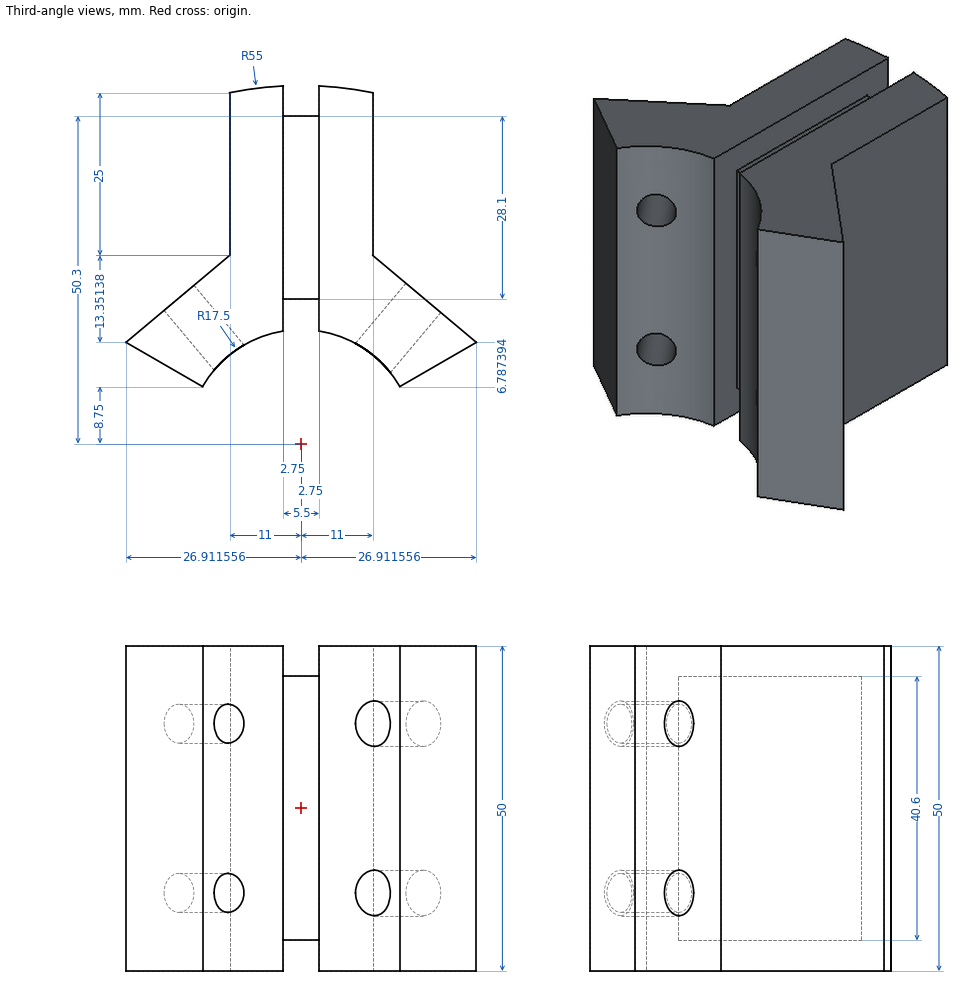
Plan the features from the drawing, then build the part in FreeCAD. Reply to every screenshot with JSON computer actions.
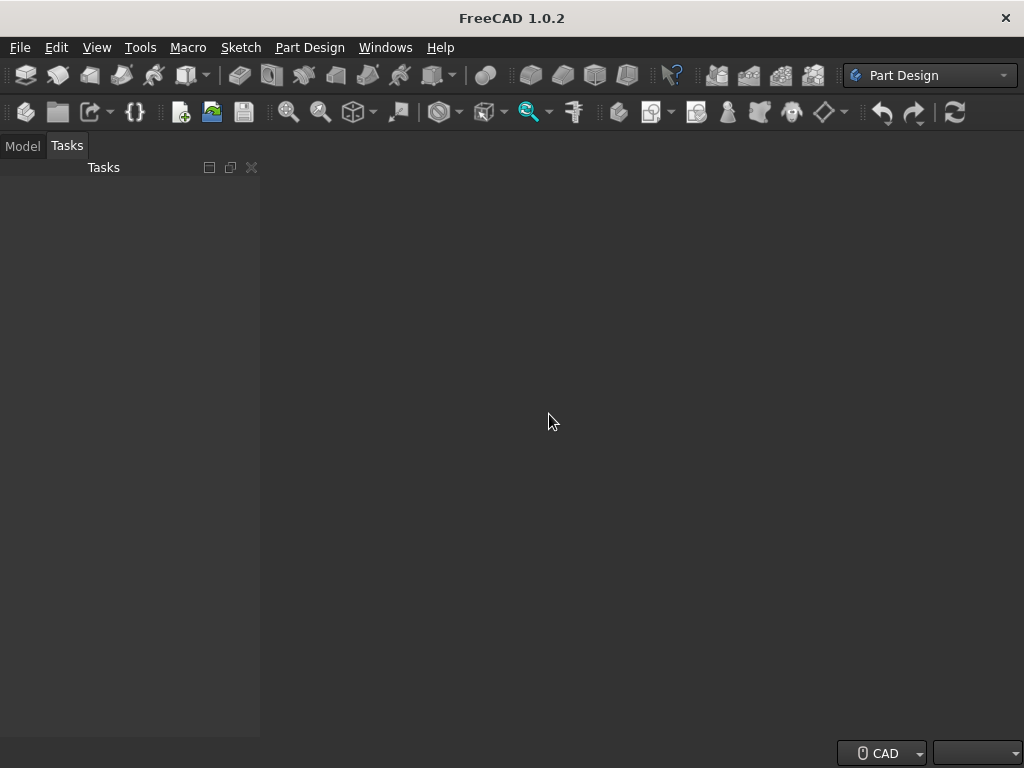
{"action": "left_click", "coordinate": [180, 112]}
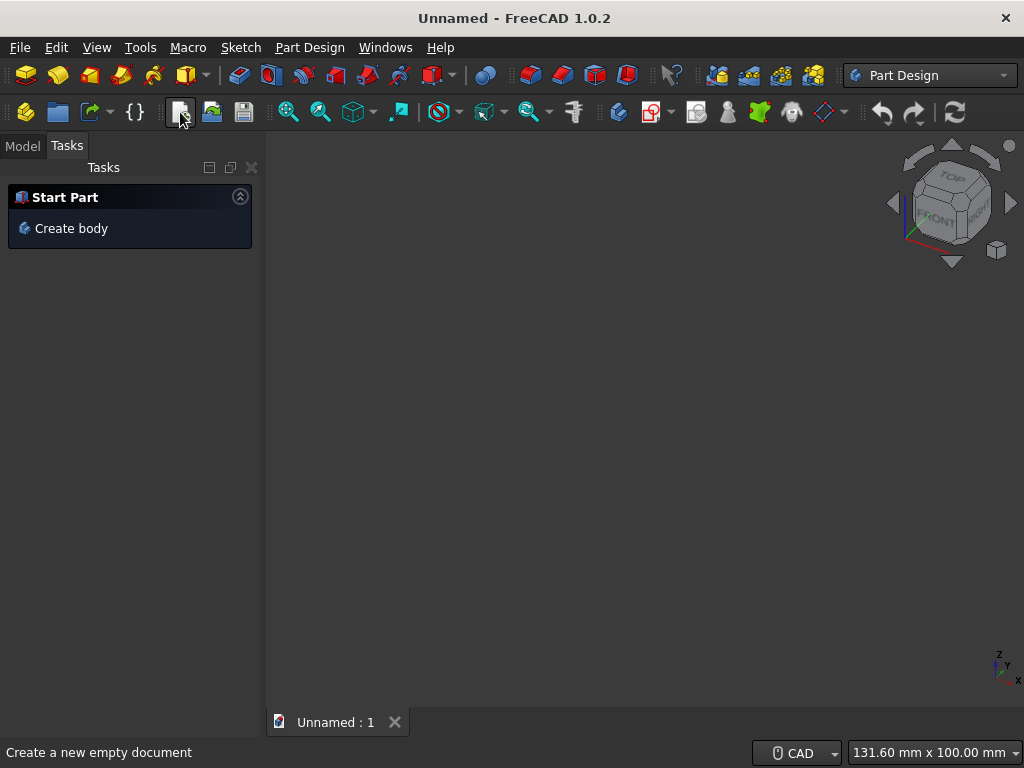
{"action": "left_click", "coordinate": [652, 112]}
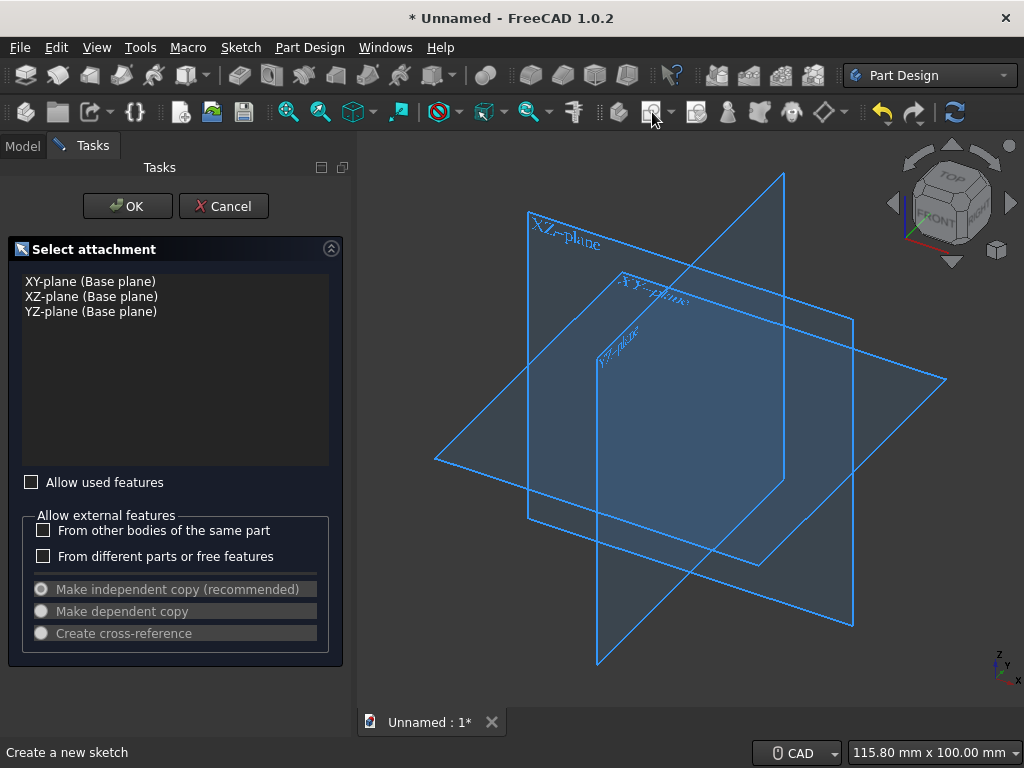
{"action": "left_click", "coordinate": [82, 282]}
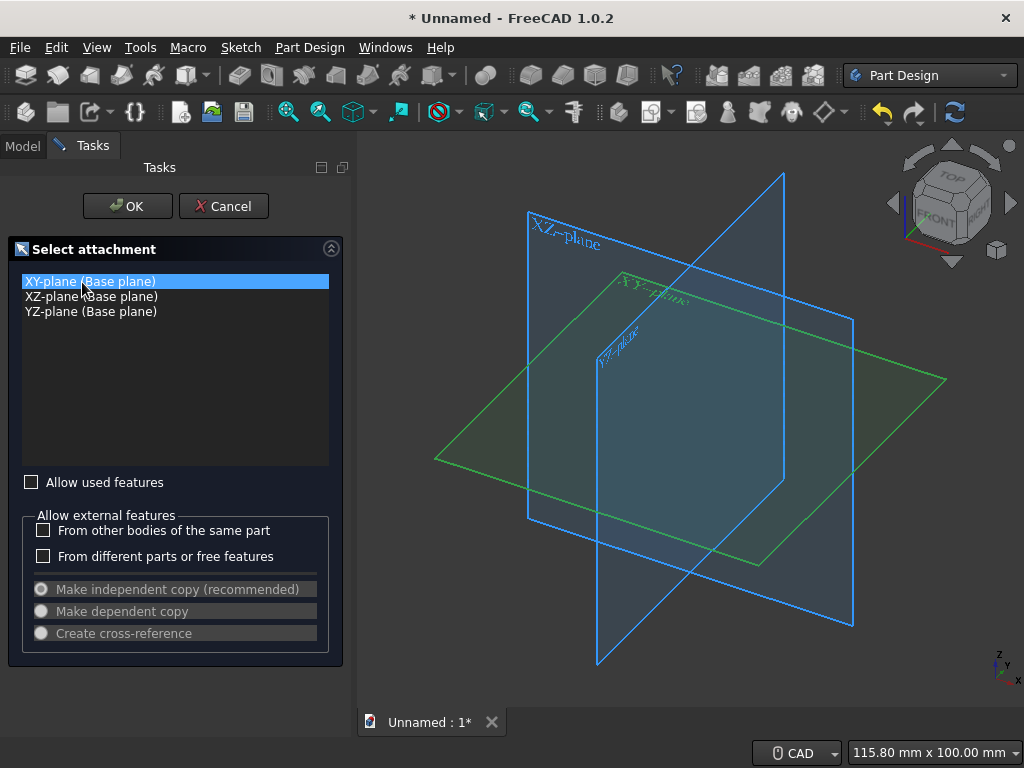
{"action": "left_click", "coordinate": [128, 206]}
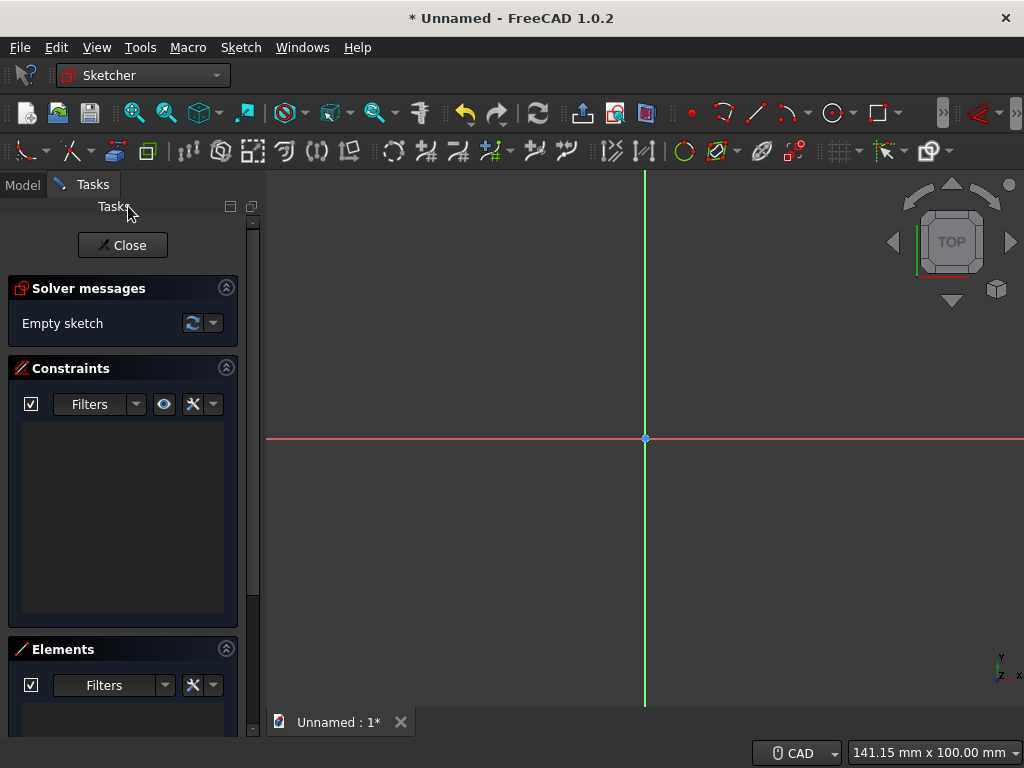
{"action": "scroll", "coordinate": [593, 679], "scroll_direction": "down", "scroll_amount": 1}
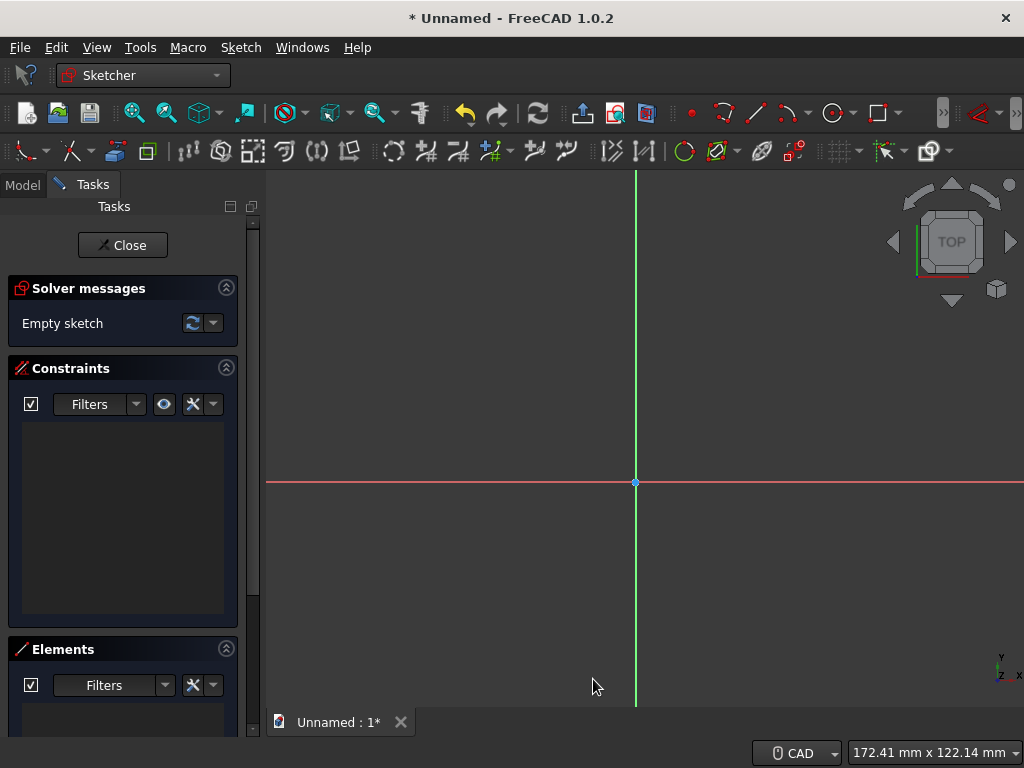
{"action": "scroll", "coordinate": [576, 205], "scroll_direction": "up", "scroll_amount": 2}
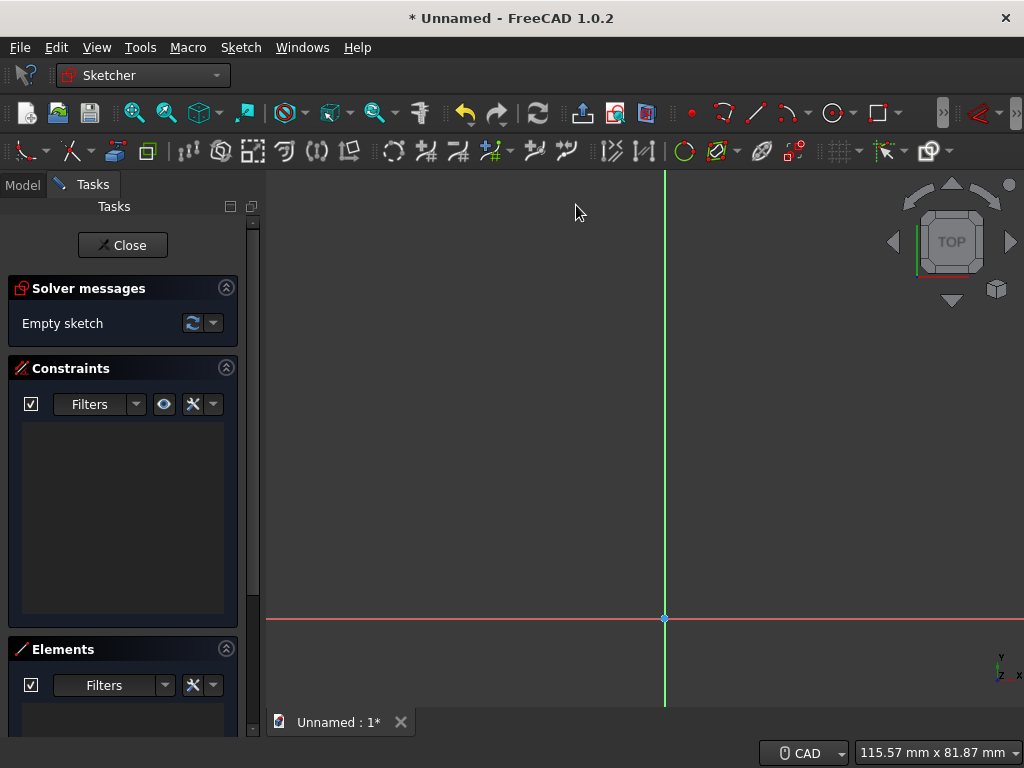
{"action": "left_click", "coordinate": [756, 114]}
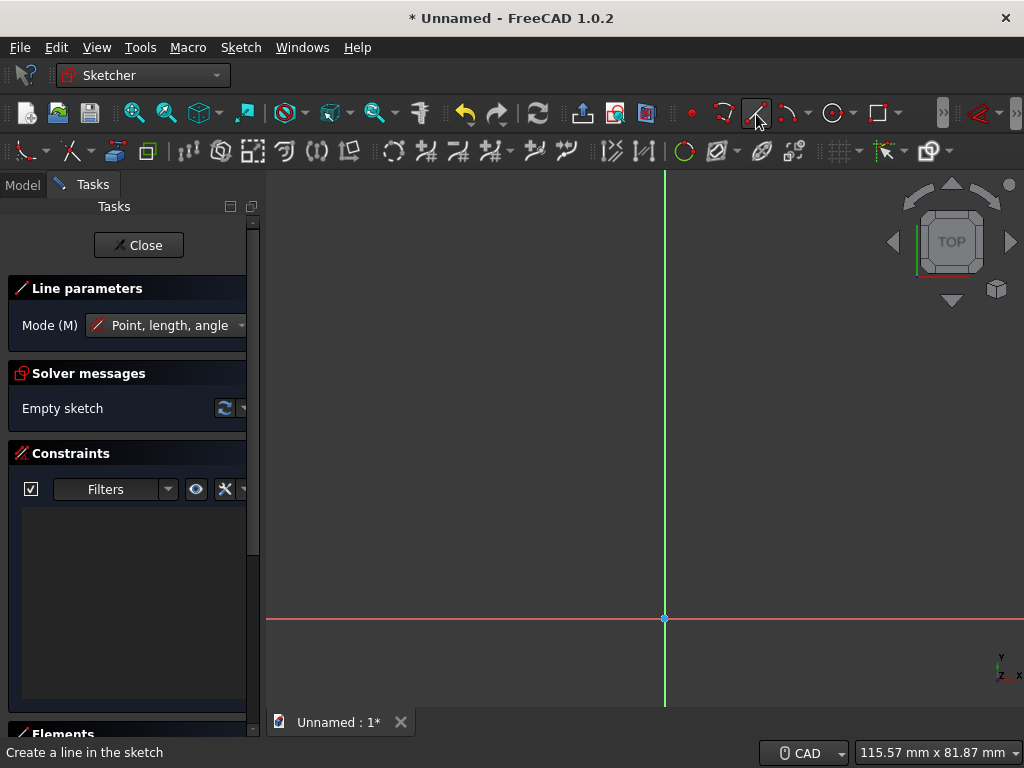
{"action": "left_click", "coordinate": [647, 505]}
{"action": "left_click", "coordinate": [647, 258]}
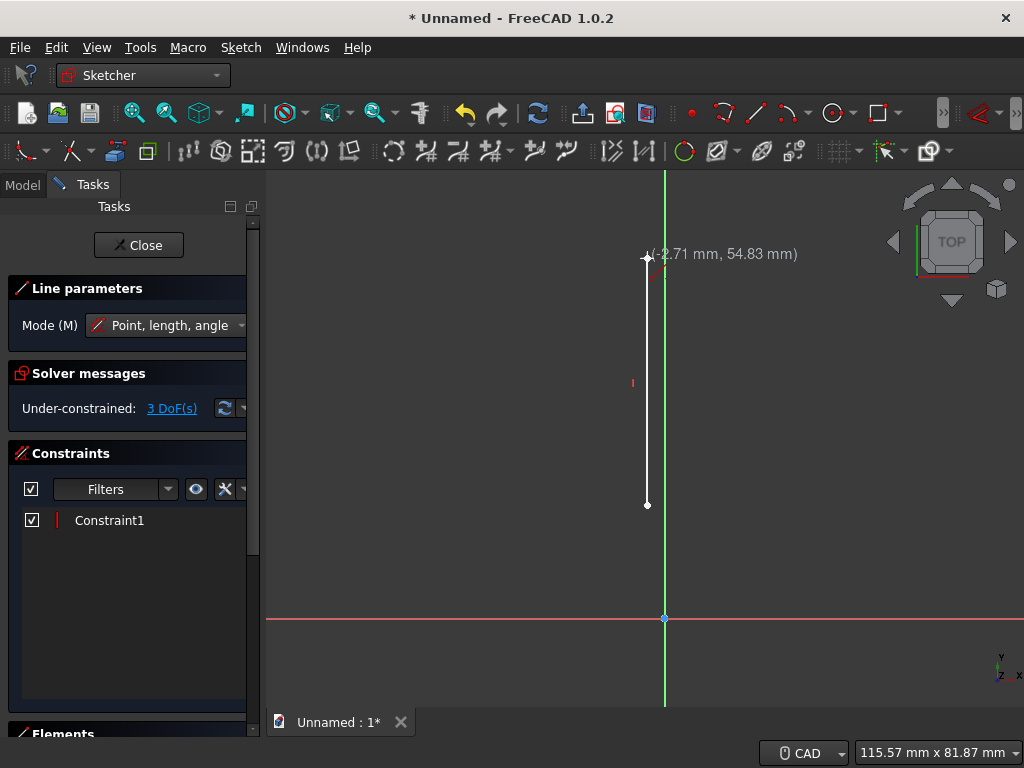
{"action": "left_click", "coordinate": [724, 114]}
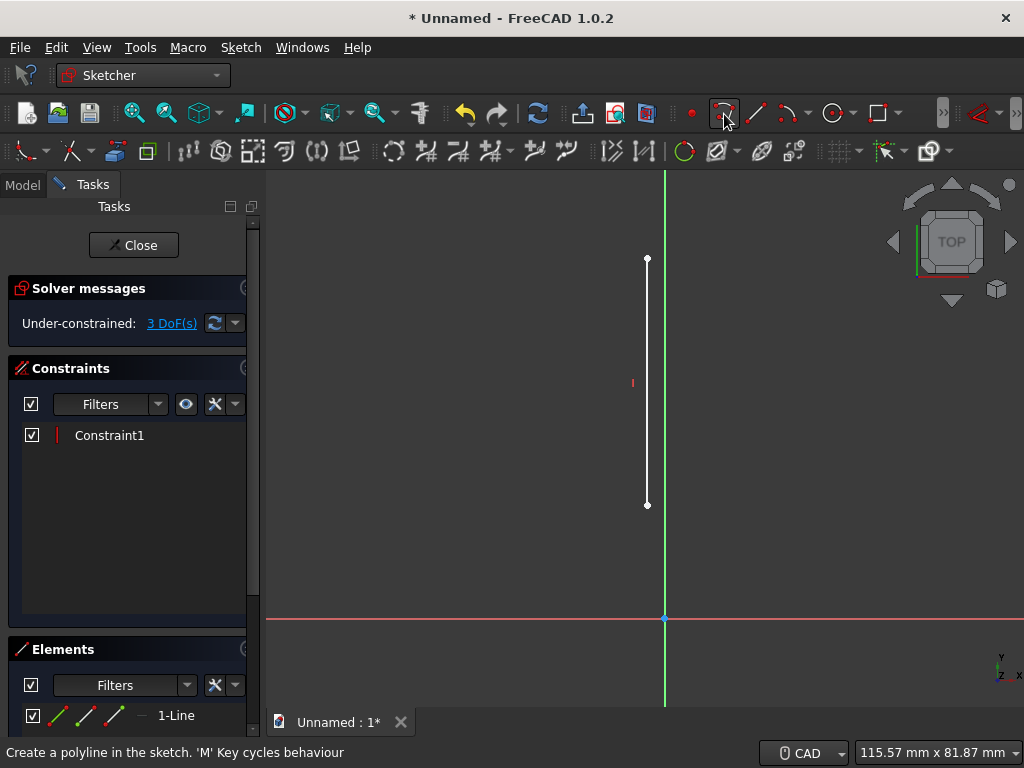
{"action": "left_click", "coordinate": [593, 265]}
{"action": "left_click", "coordinate": [593, 429]}
{"action": "left_click", "coordinate": [488, 517]}
{"action": "left_click", "coordinate": [565, 561]}
{"action": "right_click", "coordinate": [565, 561]}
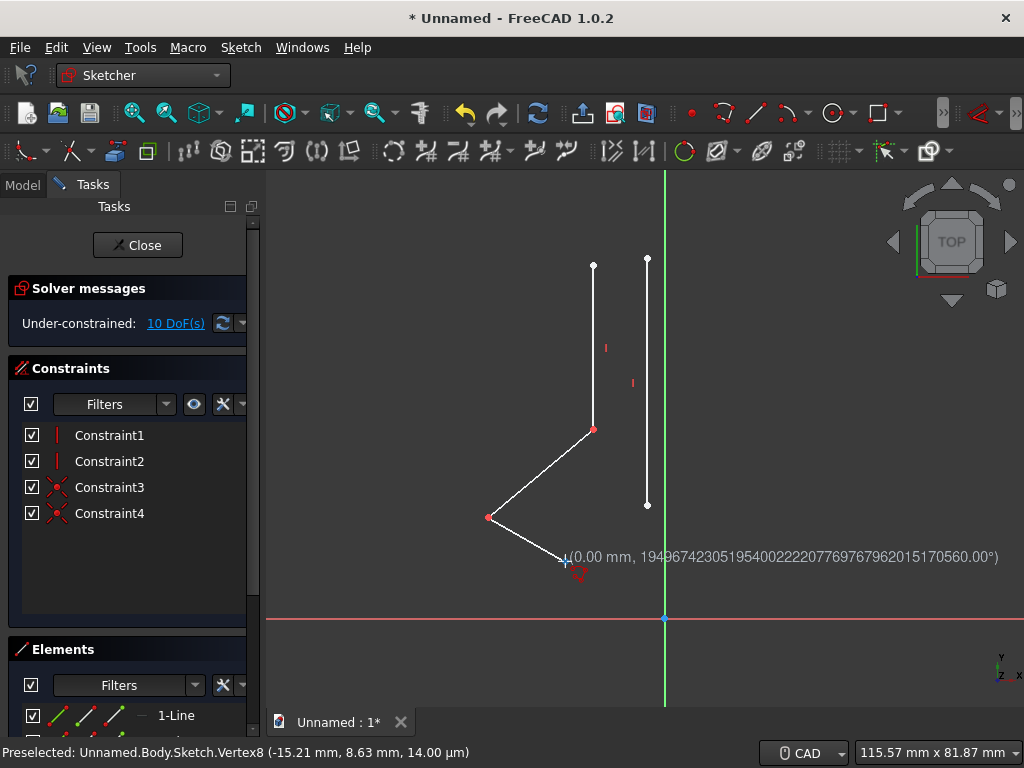
{"action": "key", "text": "g 3 a"}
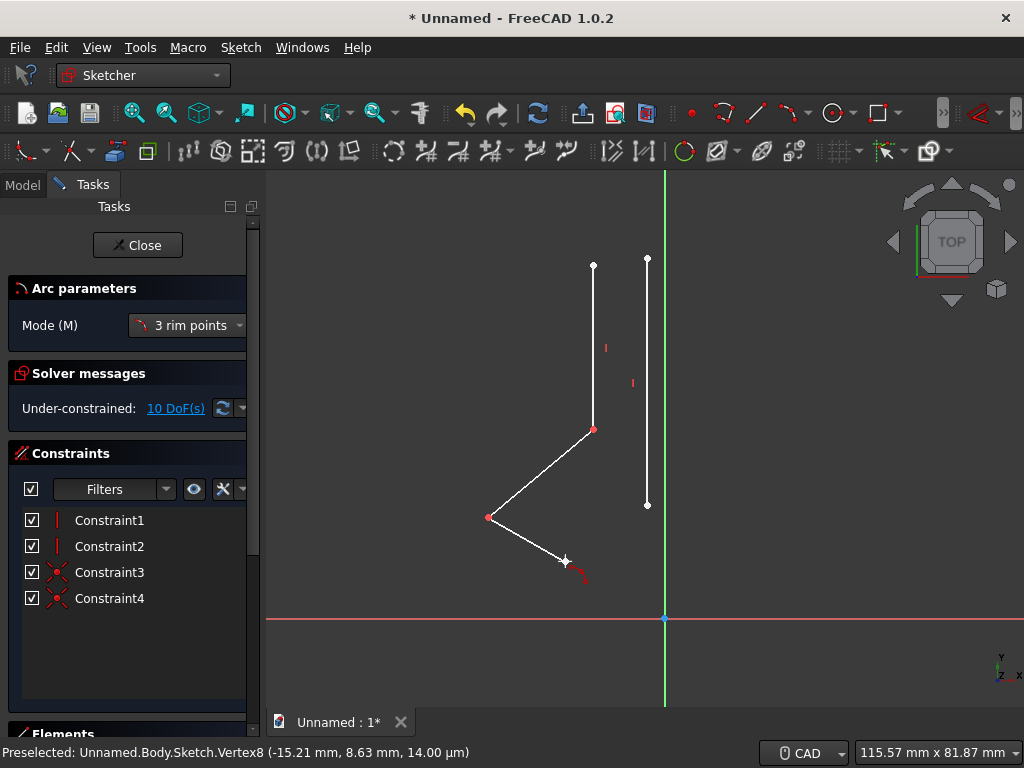
{"action": "left_click", "coordinate": [647, 259]}
{"action": "left_click", "coordinate": [593, 266]}